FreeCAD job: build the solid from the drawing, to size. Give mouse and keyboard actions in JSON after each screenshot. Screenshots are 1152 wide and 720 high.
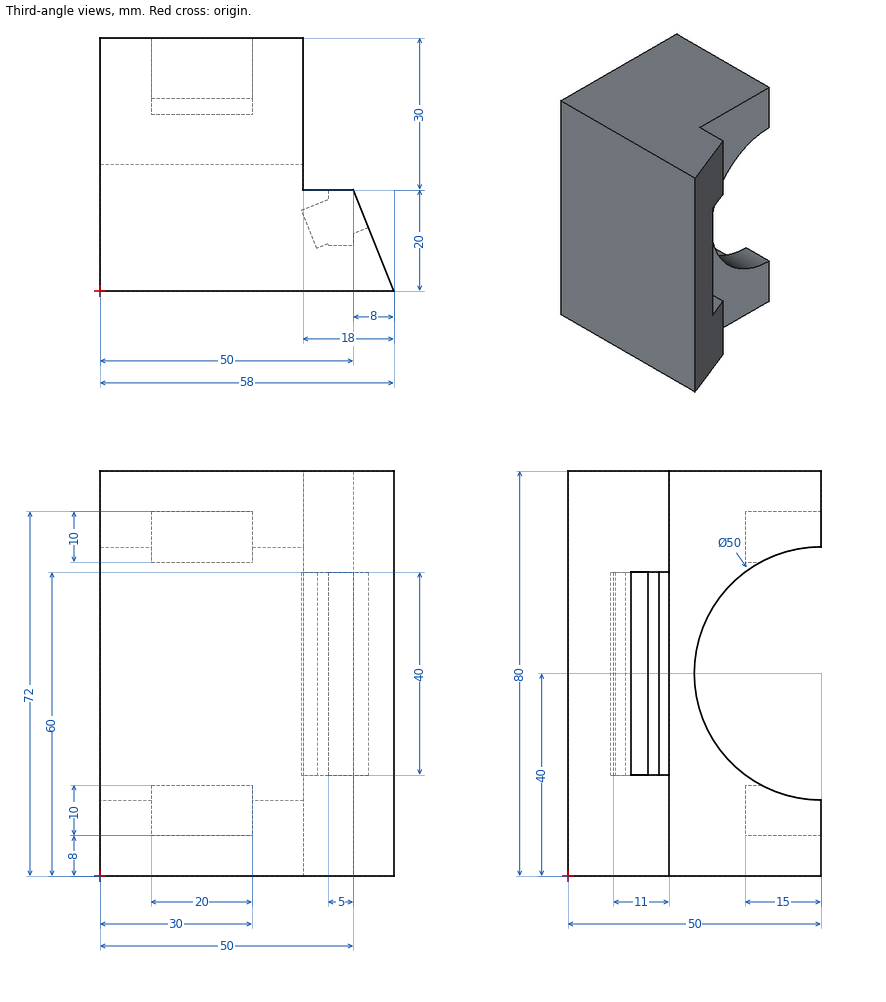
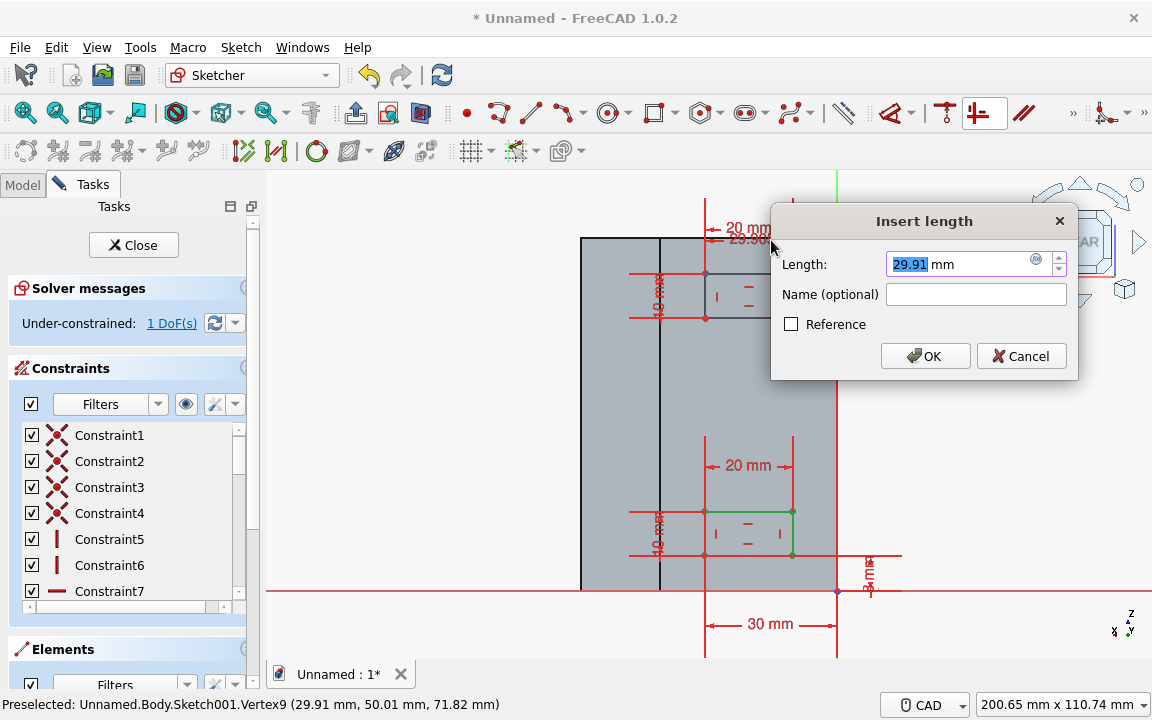
{"action": "type", "text": "30"}
{"action": "key", "text": "Return"}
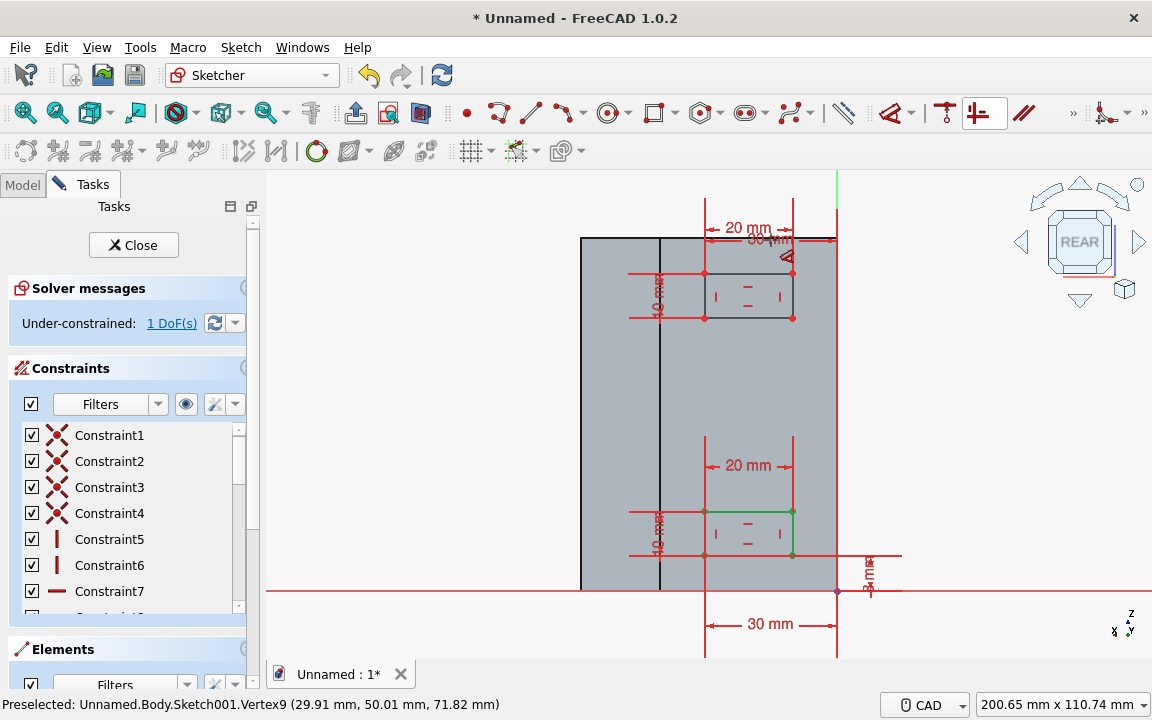
{"action": "left_click", "coordinate": [705, 274]}
{"action": "left_click", "coordinate": [871, 433]}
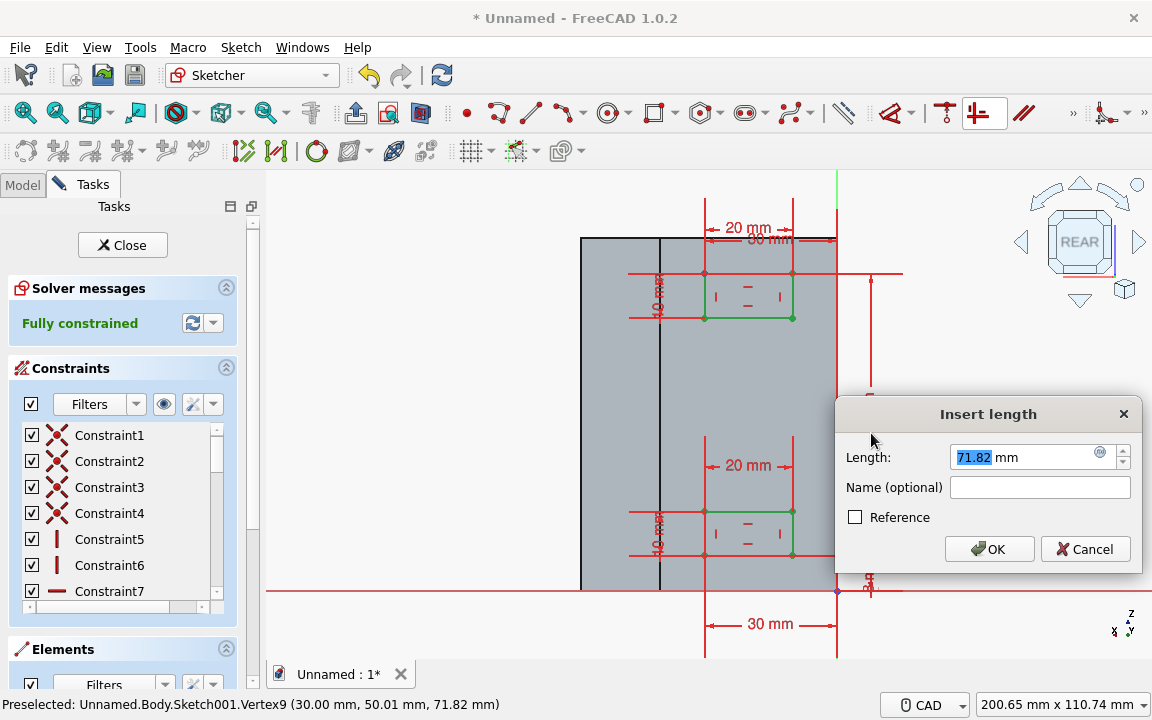
{"action": "type", "text": "72"}
{"action": "key", "text": "Return"}
{"action": "key", "text": "Escape"}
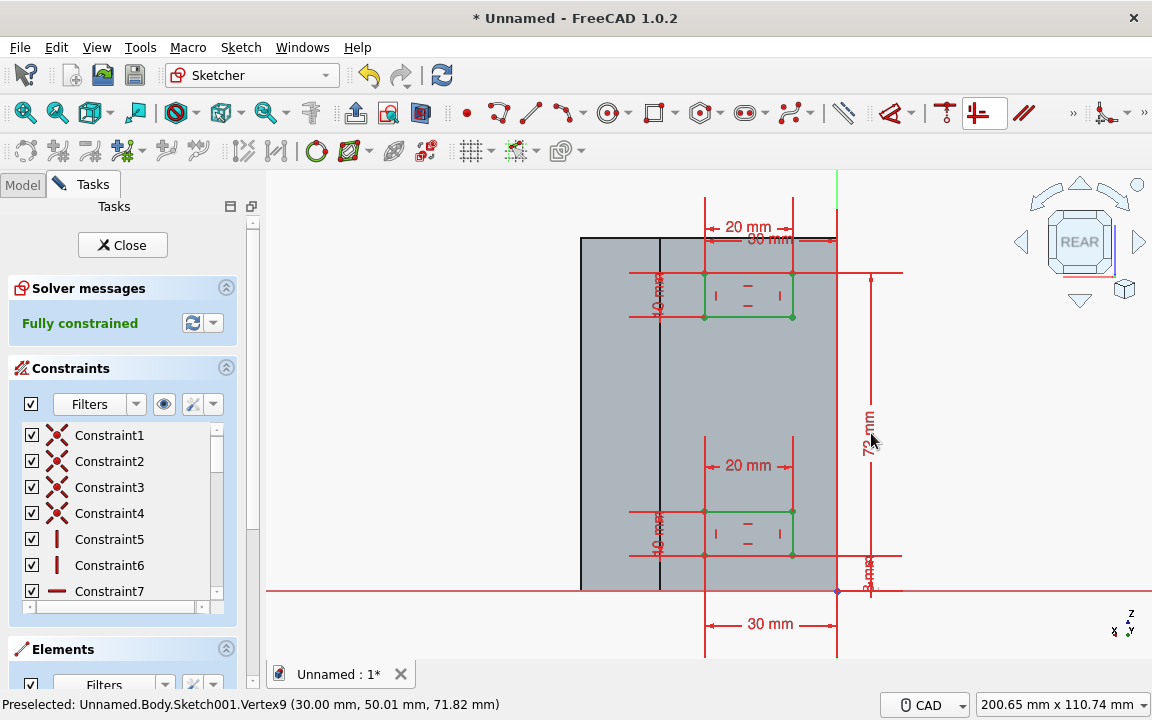
{"action": "left_click", "coordinate": [123, 245]}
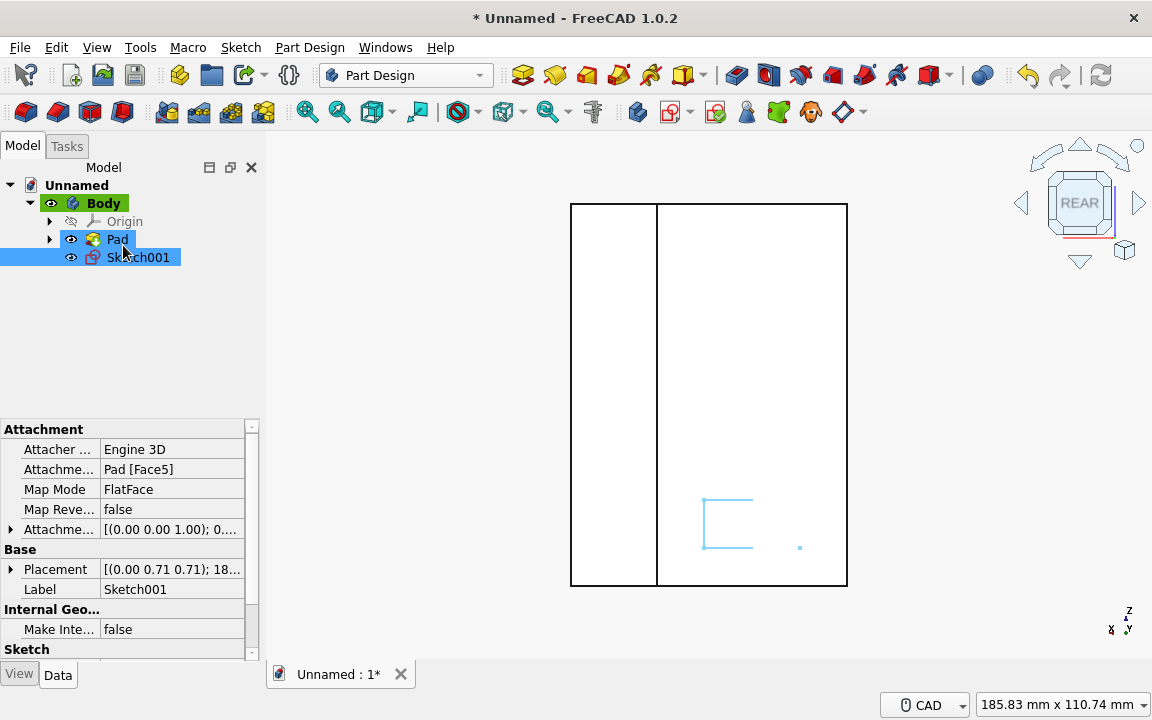
{"action": "left_click", "coordinate": [738, 76]}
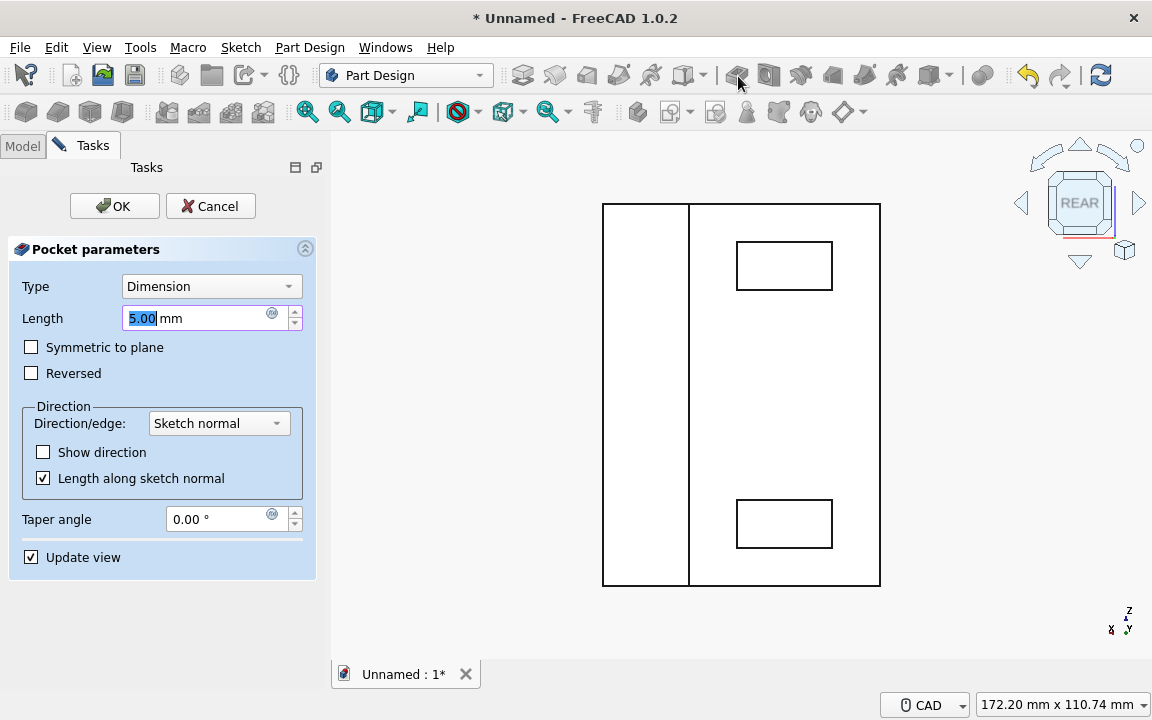
{"action": "type", "text": "15"}
{"action": "key", "text": "Tab"}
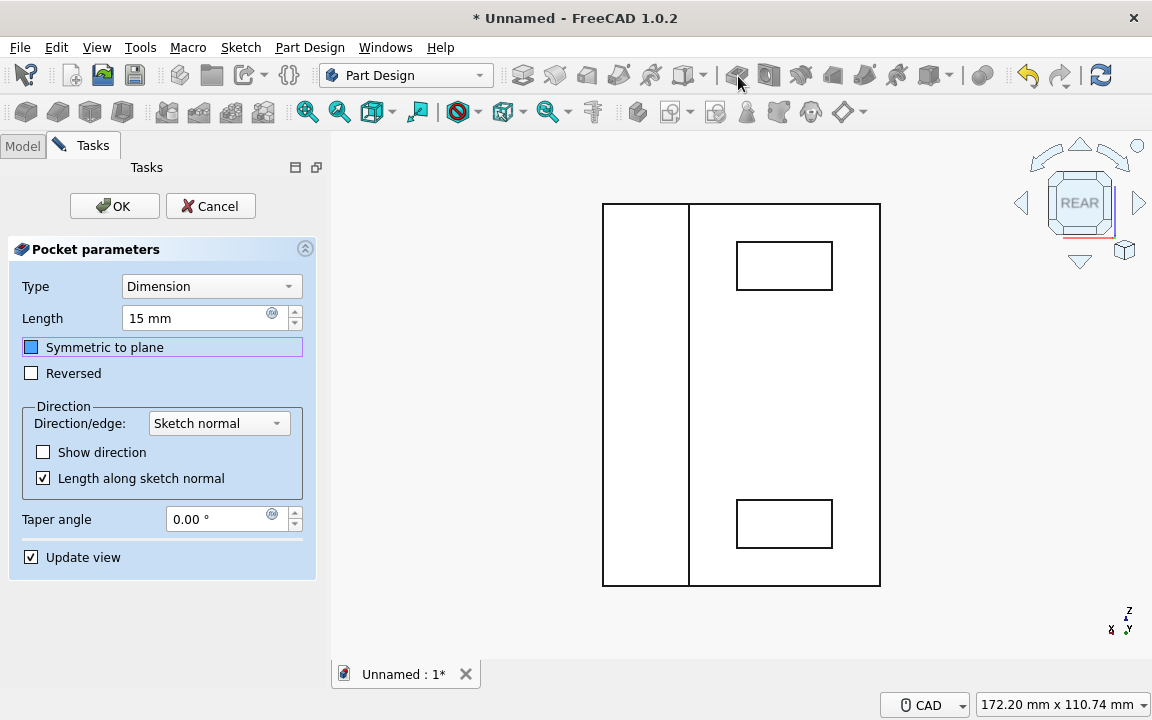
{"action": "left_click", "coordinate": [115, 206]}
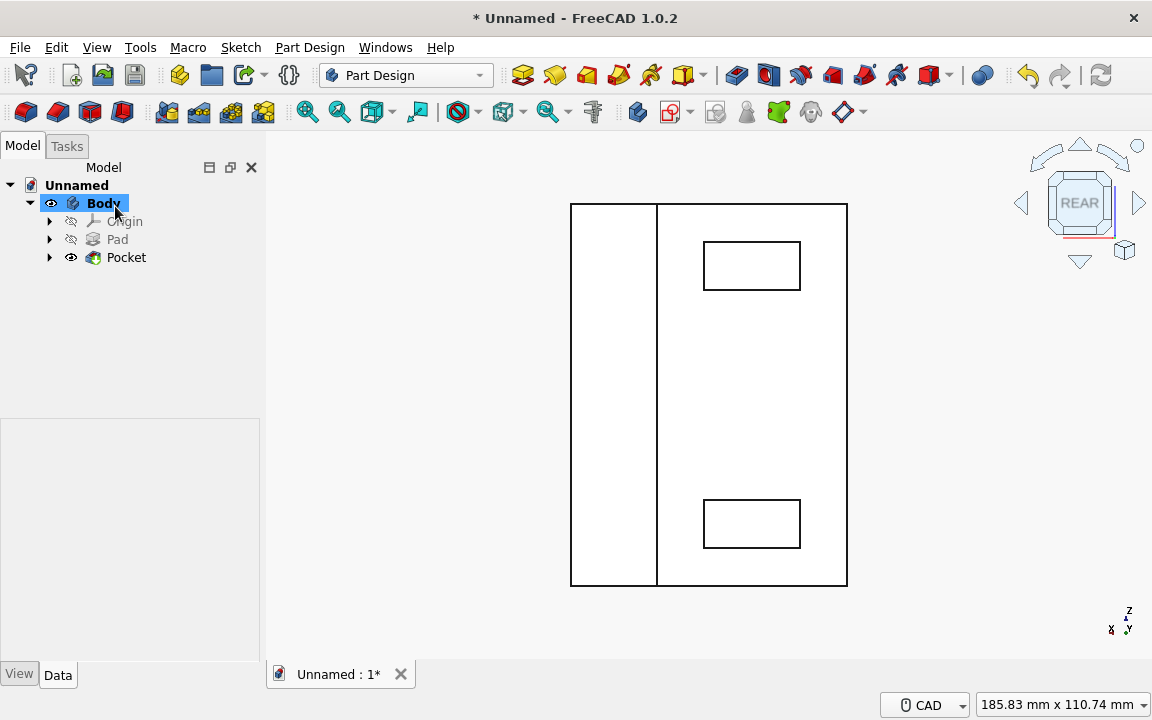
{"action": "key", "text": "0"}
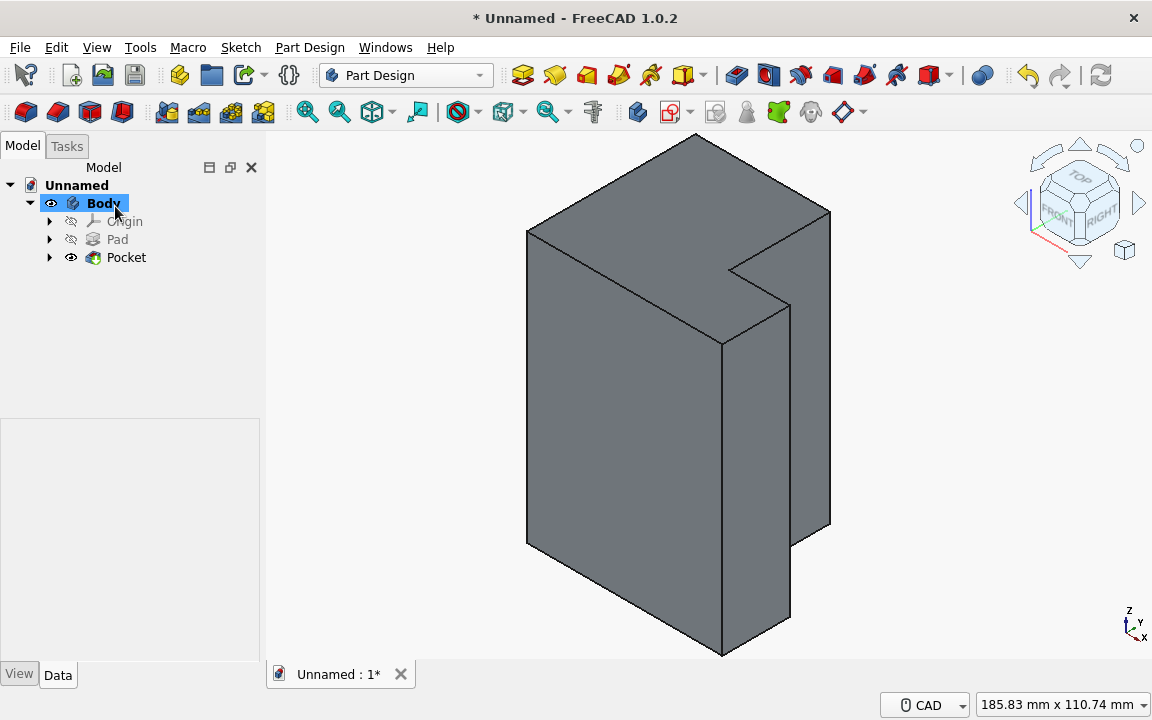
{"action": "key", "text": "3"}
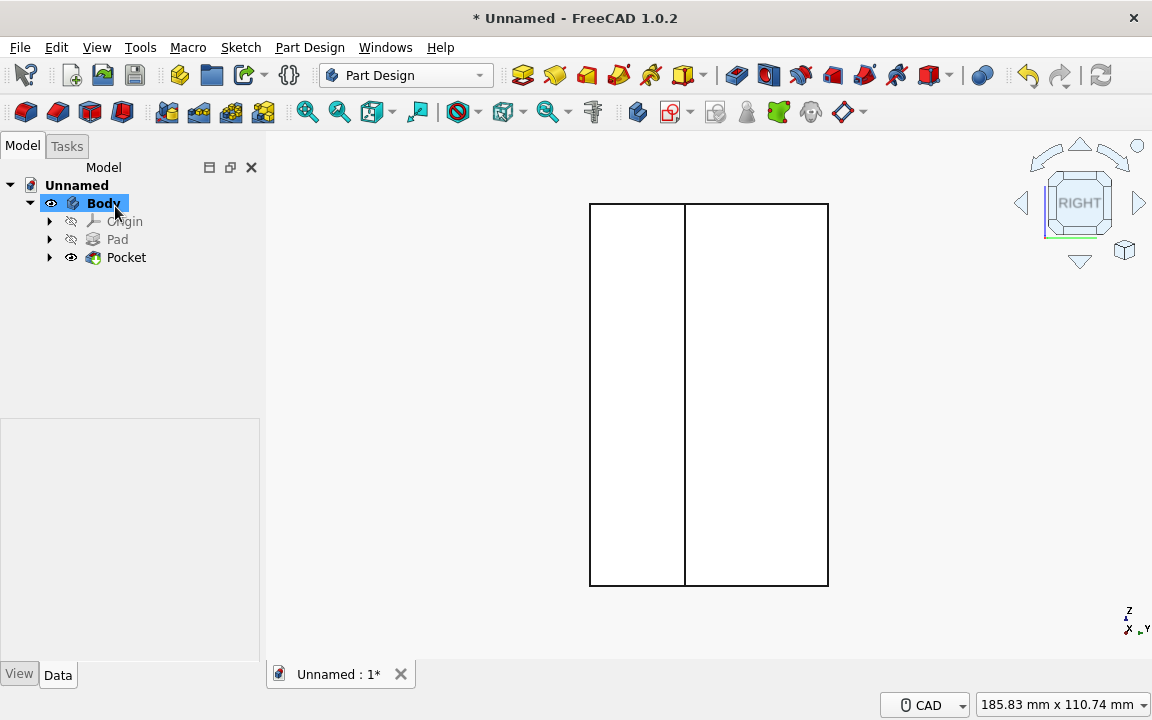
{"action": "left_click", "coordinate": [757, 285]}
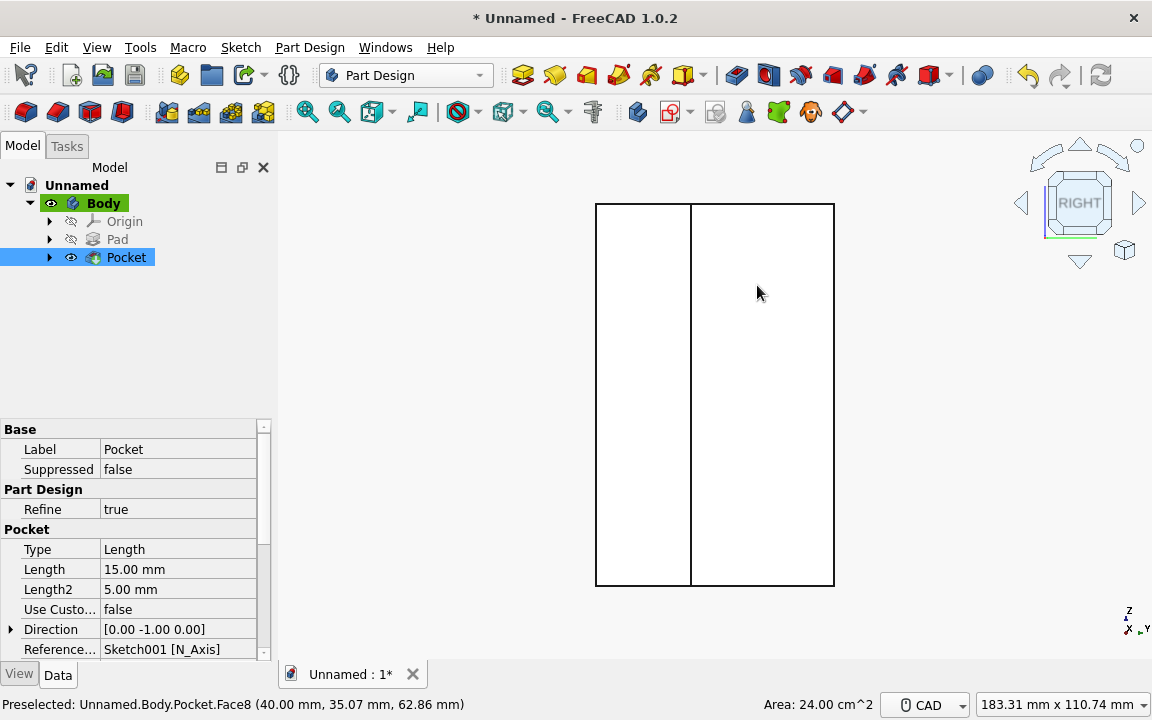
{"action": "left_click", "coordinate": [670, 112]}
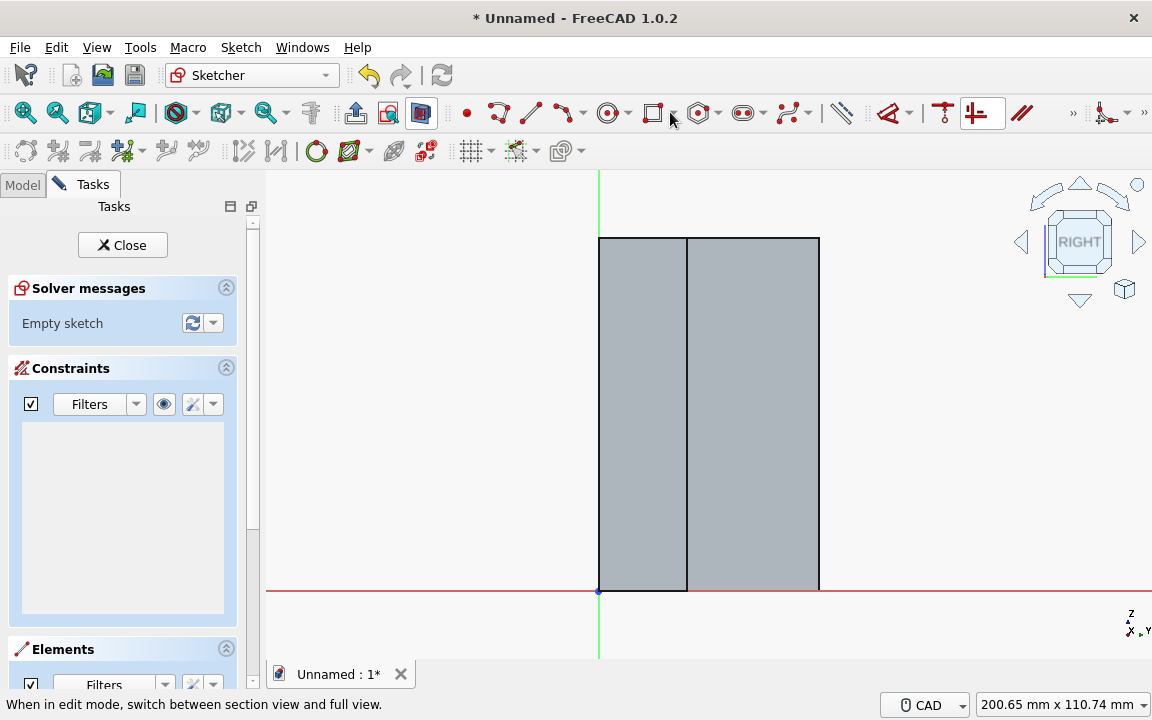
{"action": "left_click", "coordinate": [608, 114]}